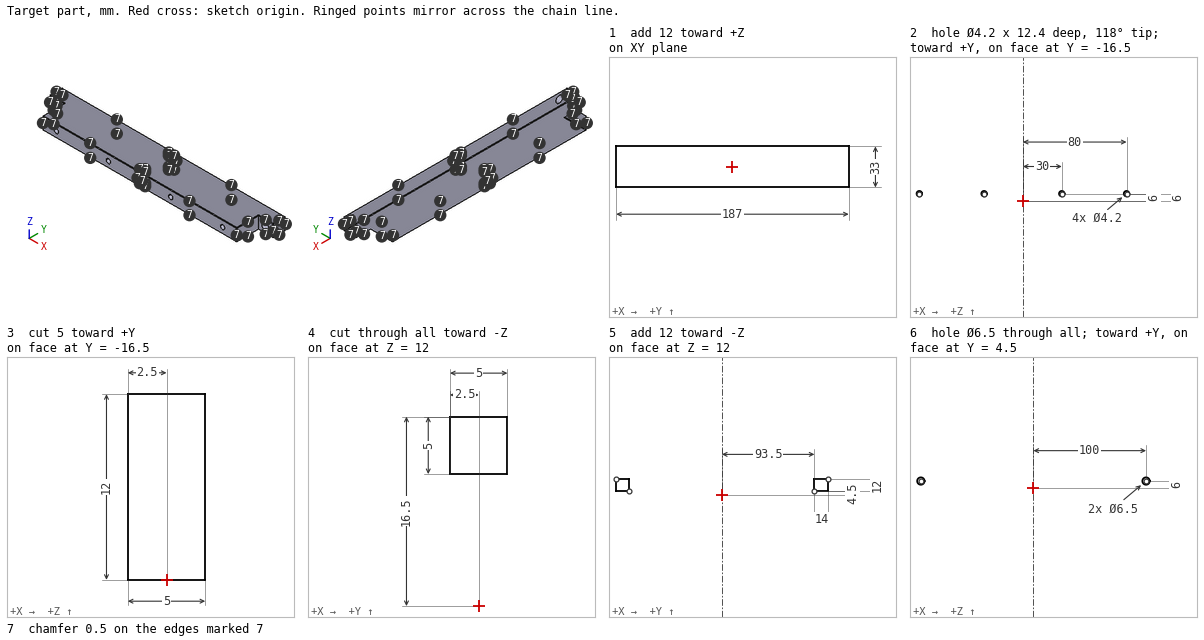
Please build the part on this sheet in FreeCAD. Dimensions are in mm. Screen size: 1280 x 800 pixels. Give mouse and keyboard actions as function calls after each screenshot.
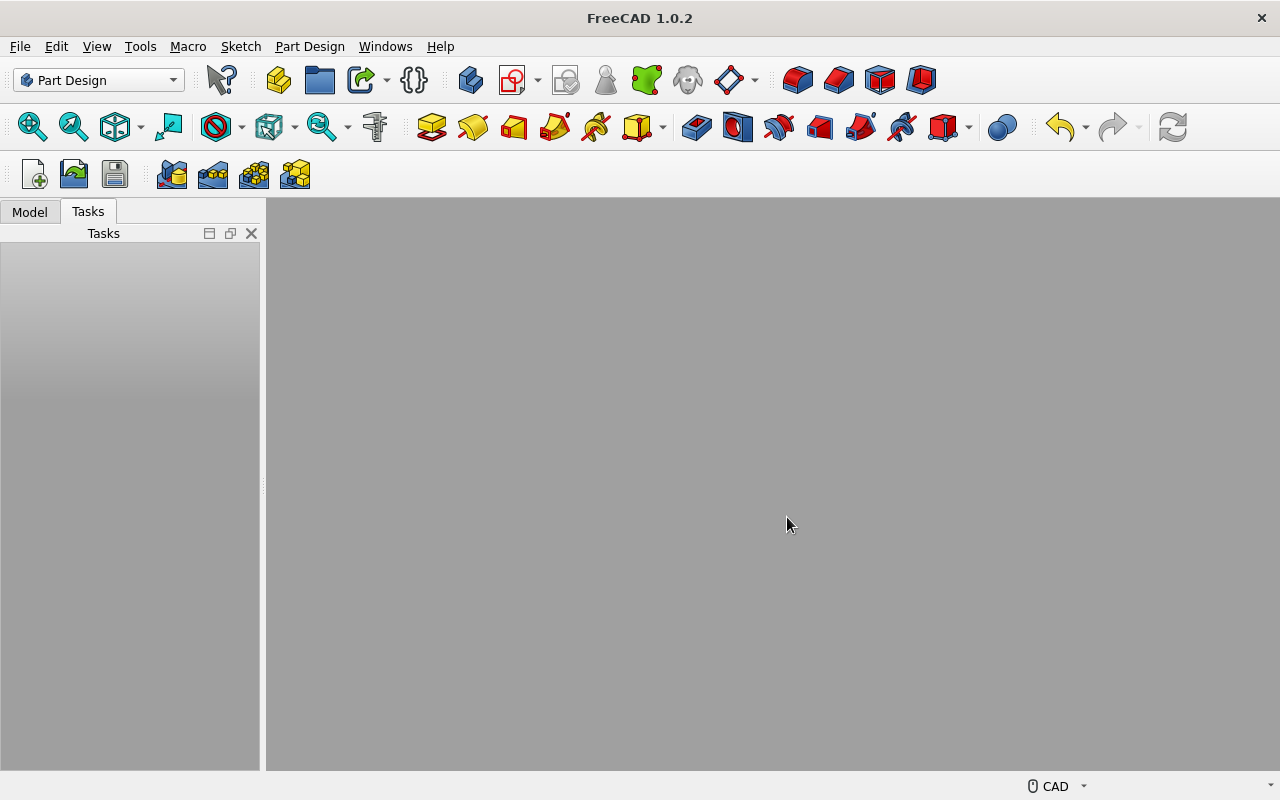
key(ctrl+n)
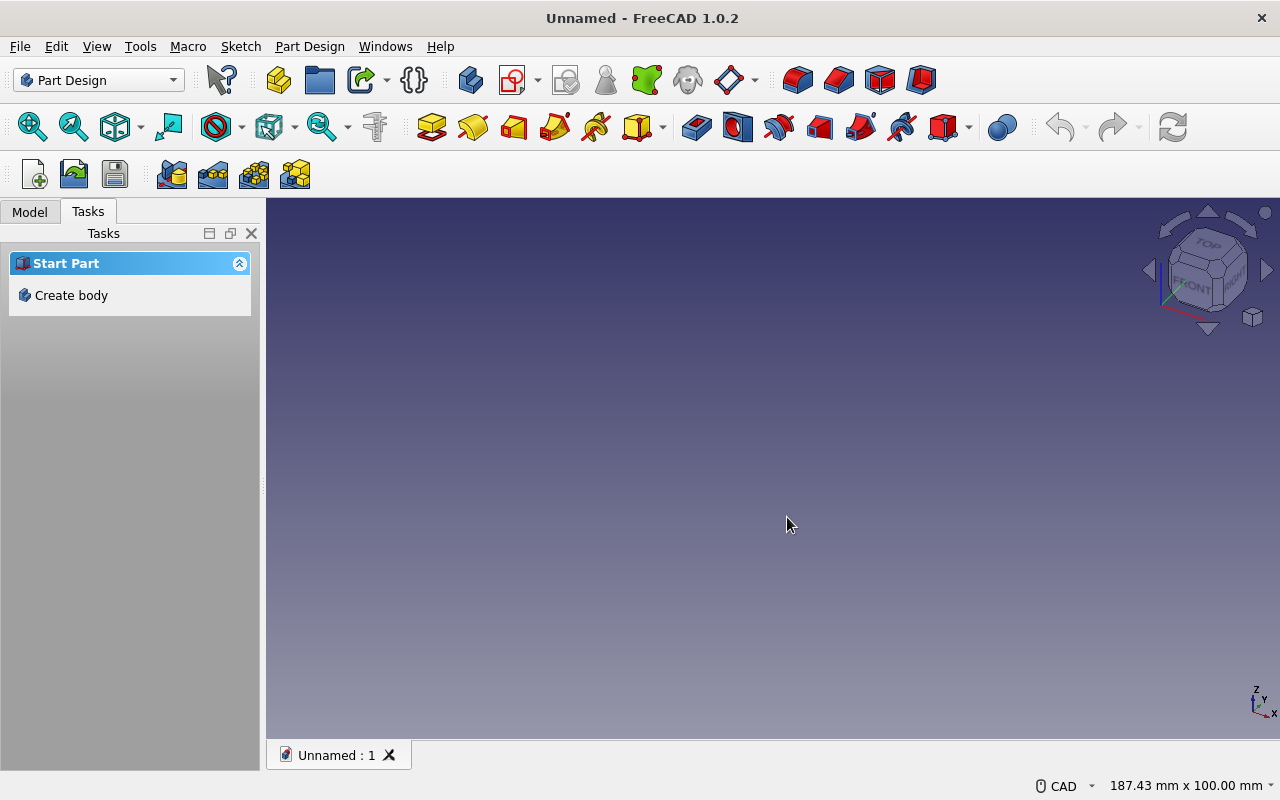
click(512, 80)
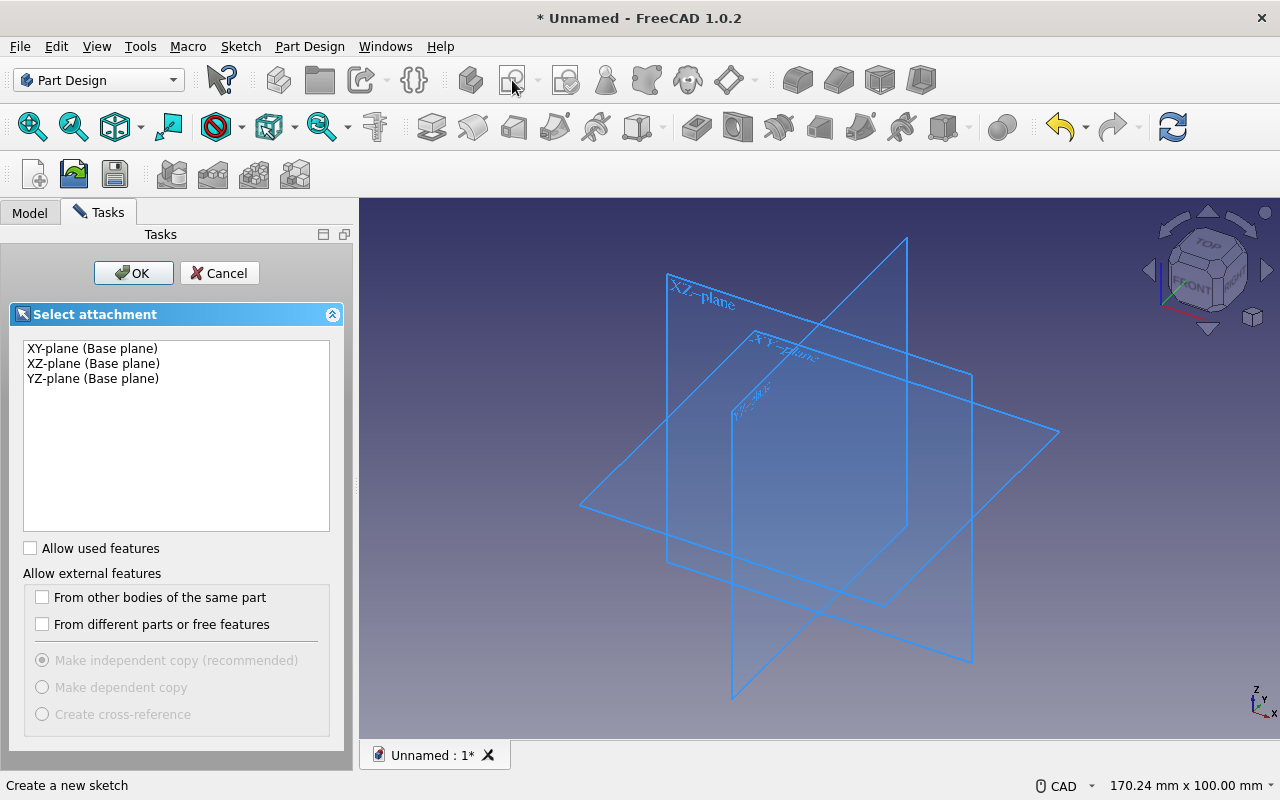
click(84, 348)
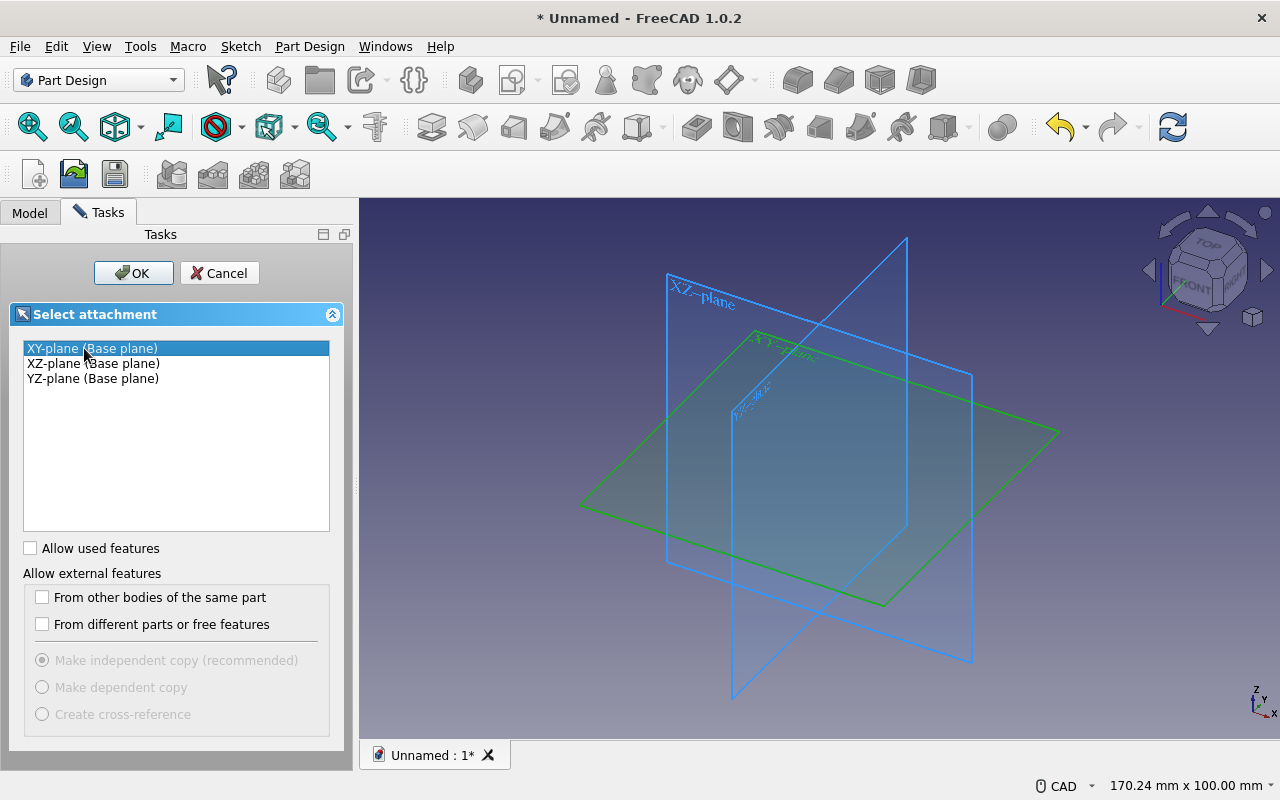
click(134, 273)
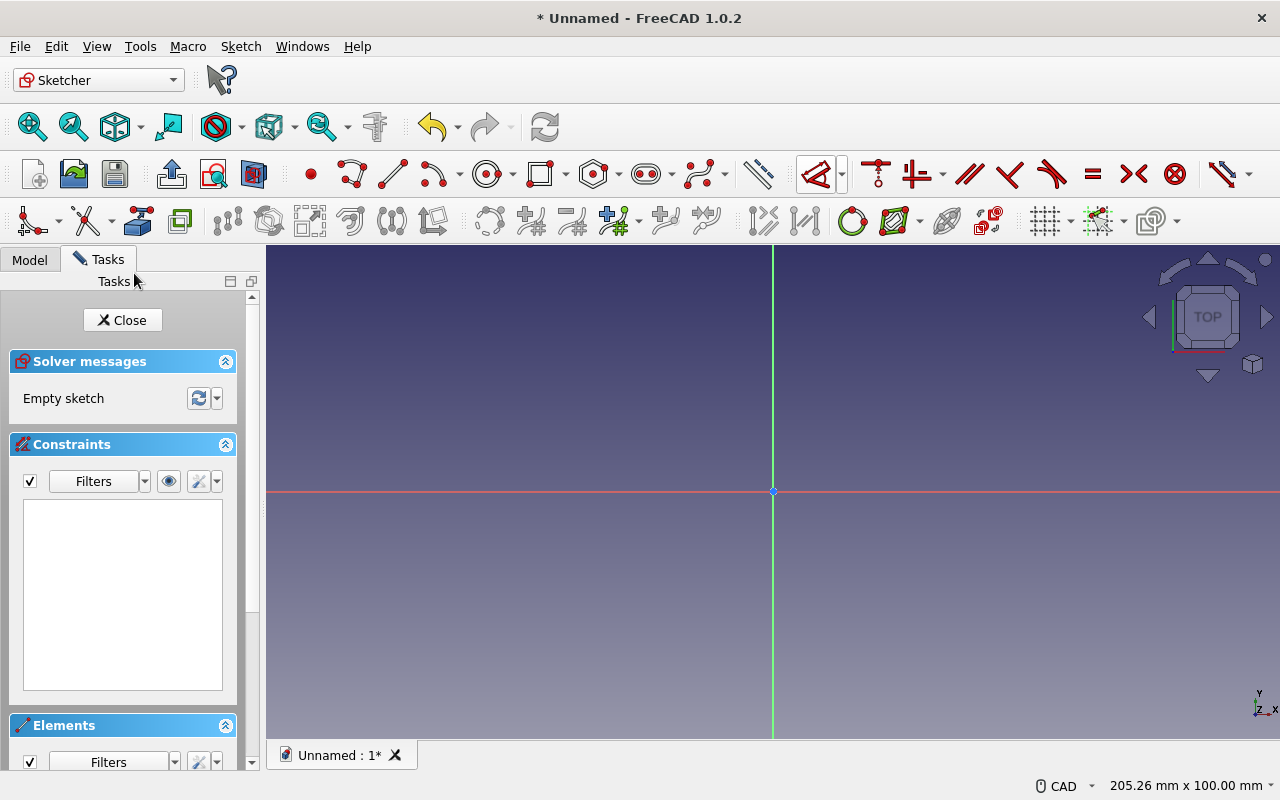
scroll(565, 492, down, 2)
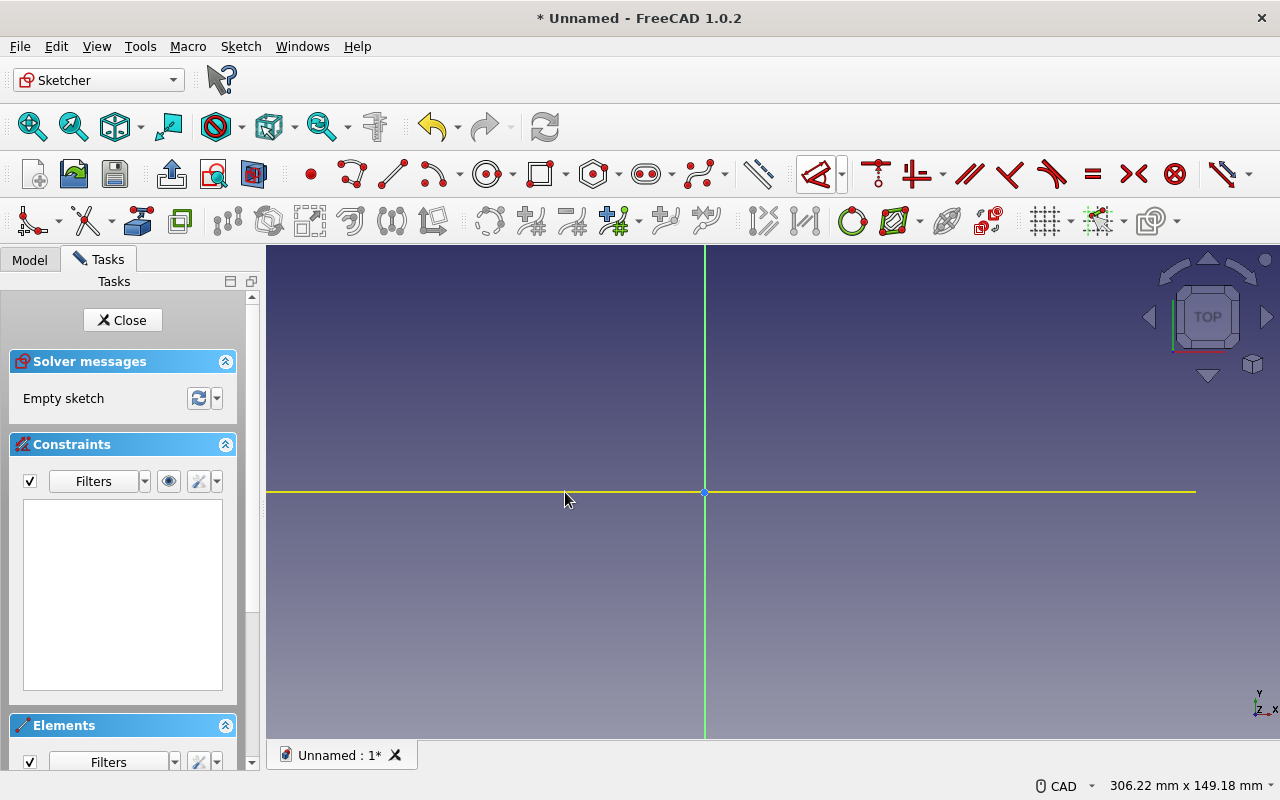
key(g)
key(v)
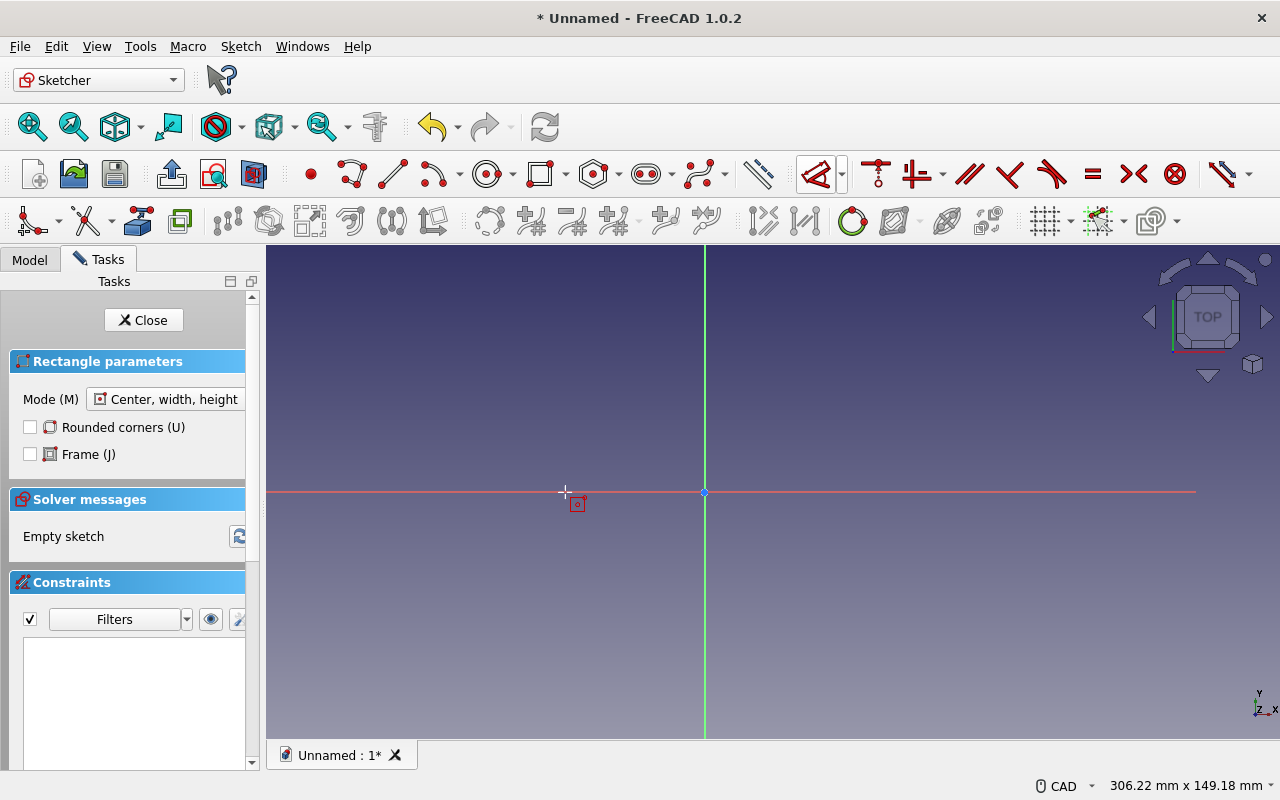
click(705, 492)
click(1014, 438)
key(Escape)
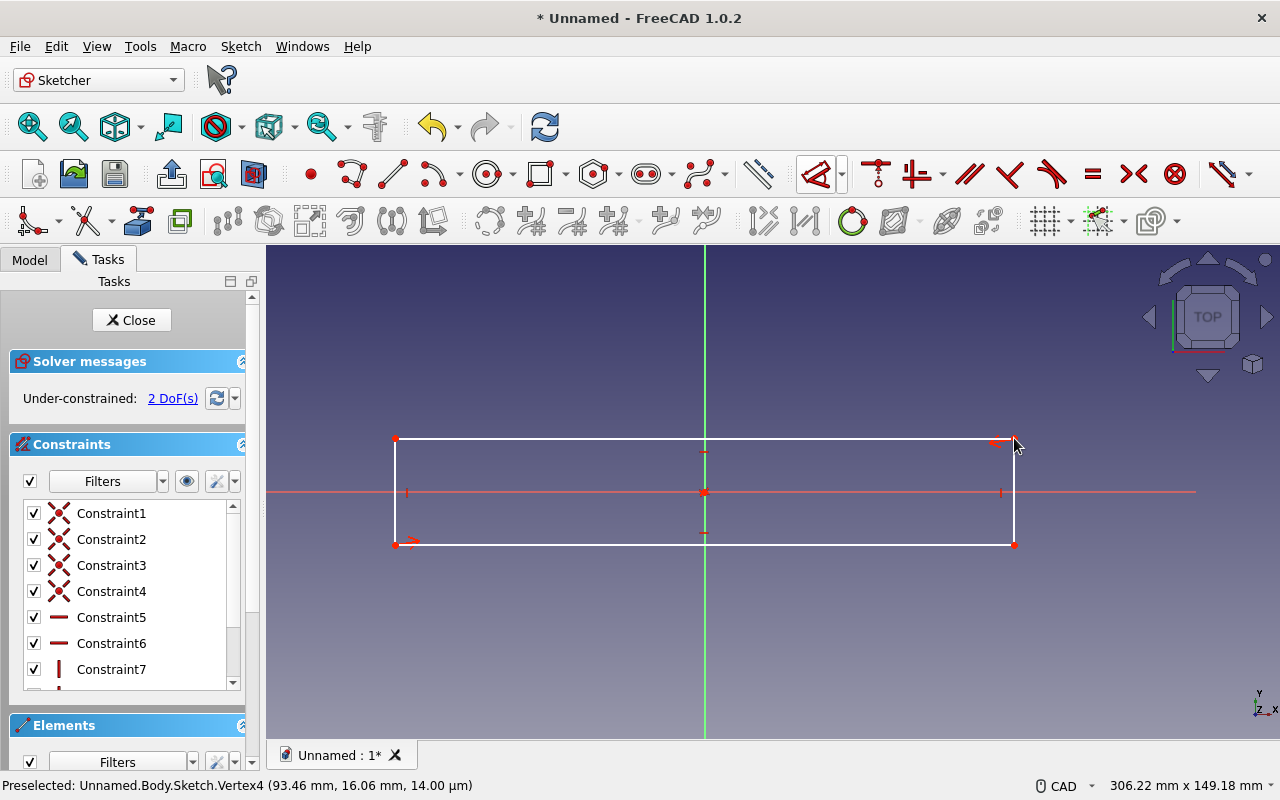
click(816, 174)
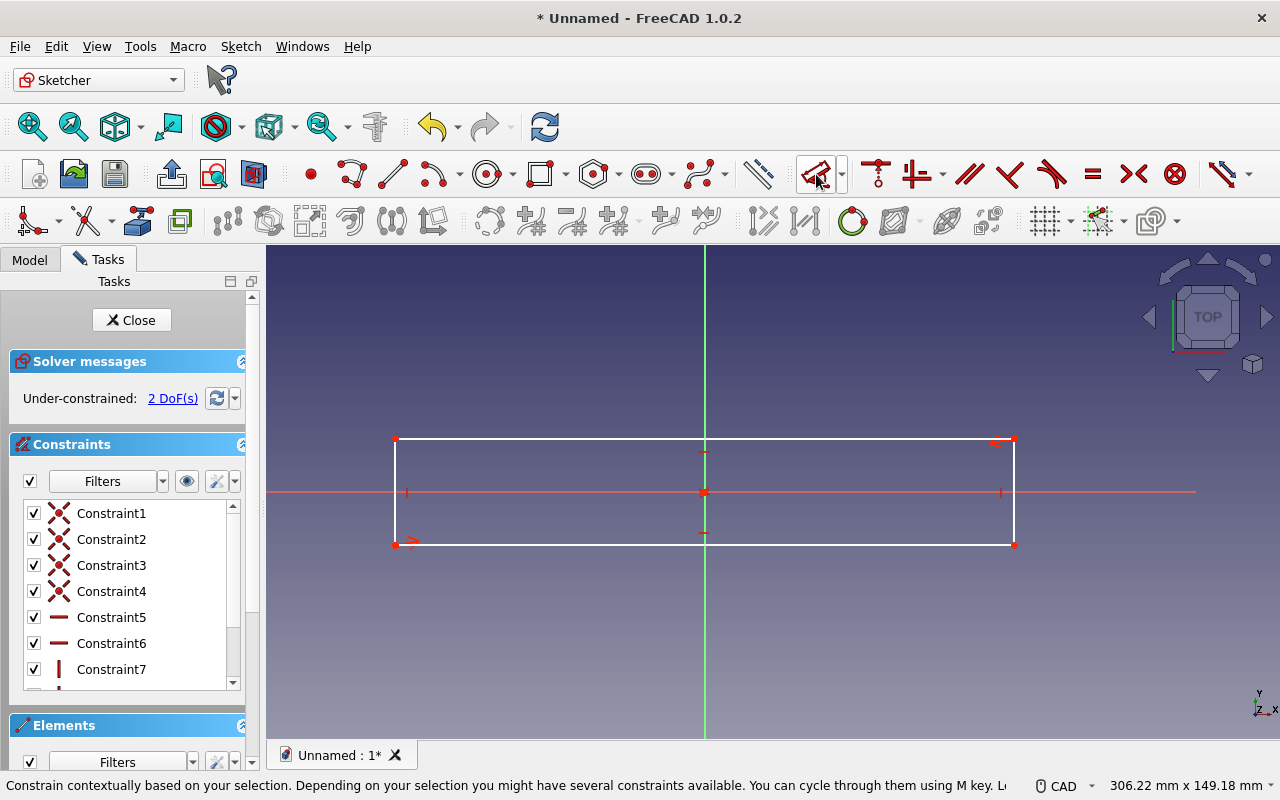
click(1014, 513)
click(1048, 468)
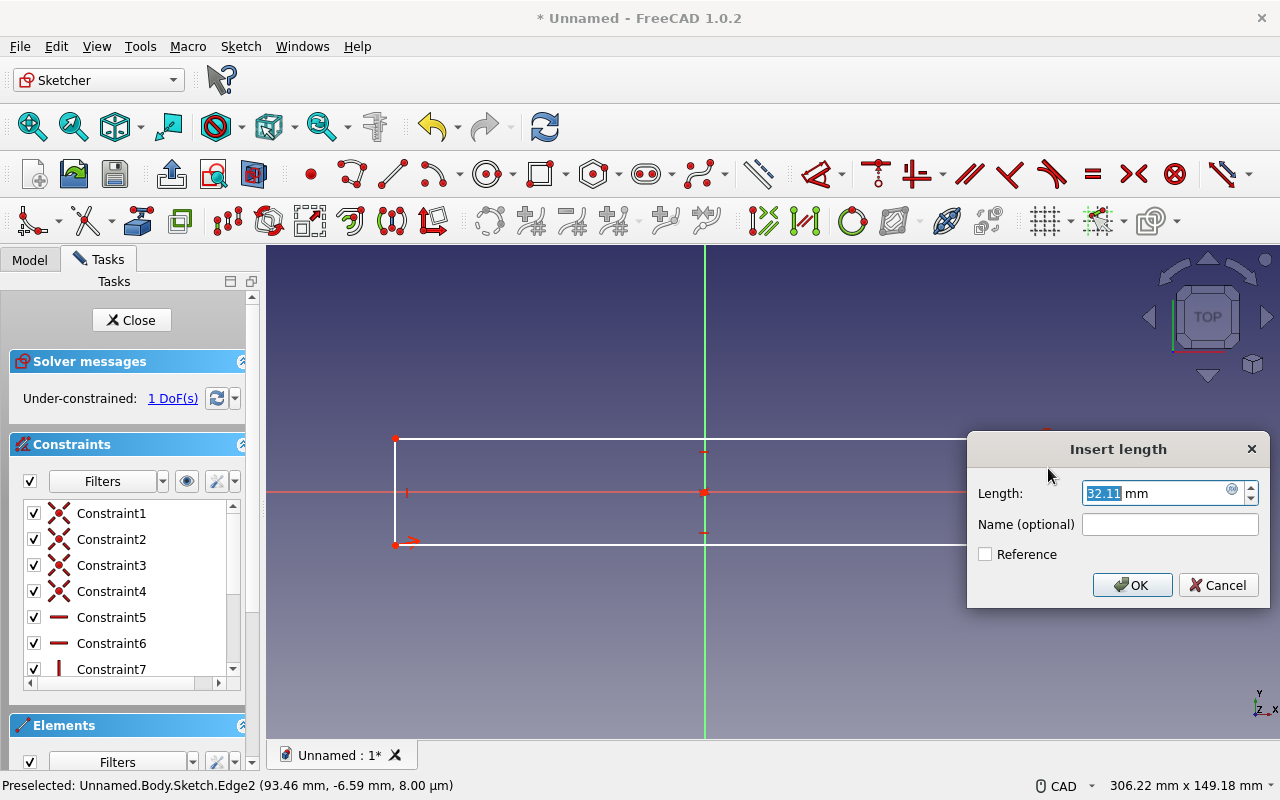
text(33)
key(Return)